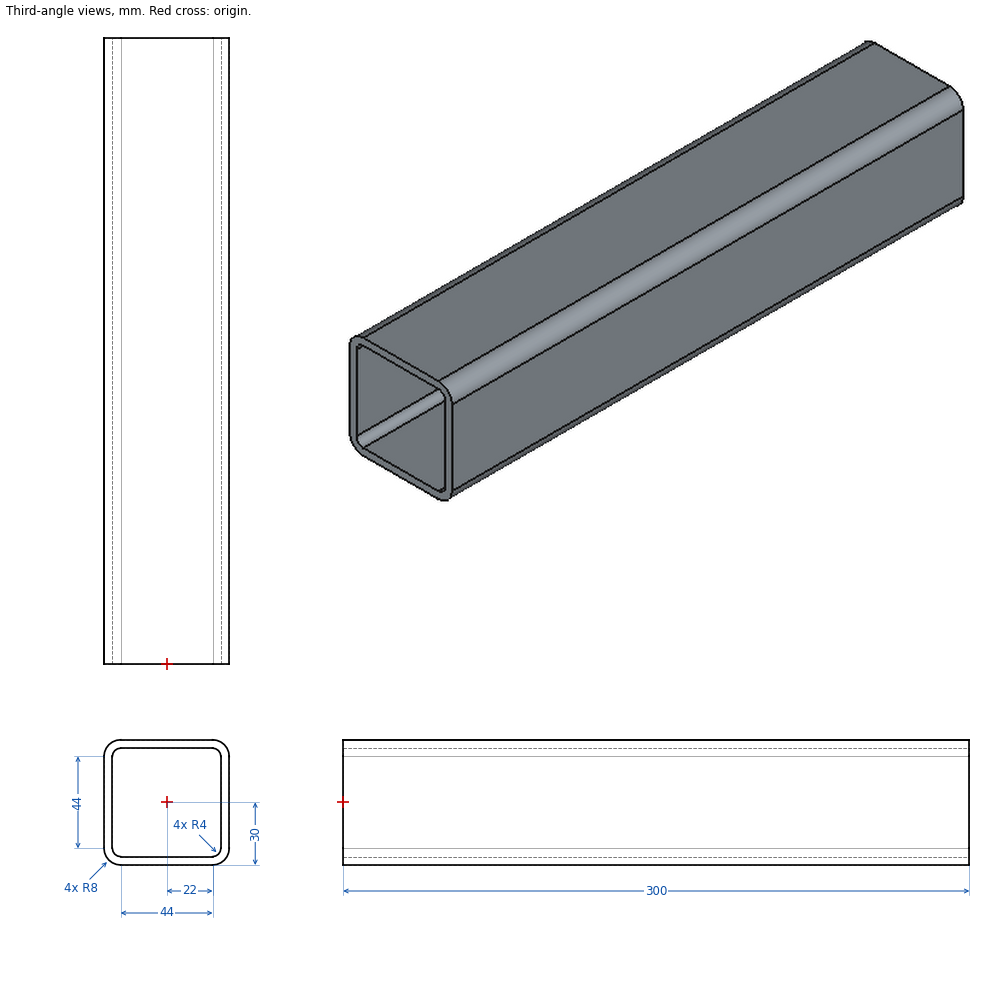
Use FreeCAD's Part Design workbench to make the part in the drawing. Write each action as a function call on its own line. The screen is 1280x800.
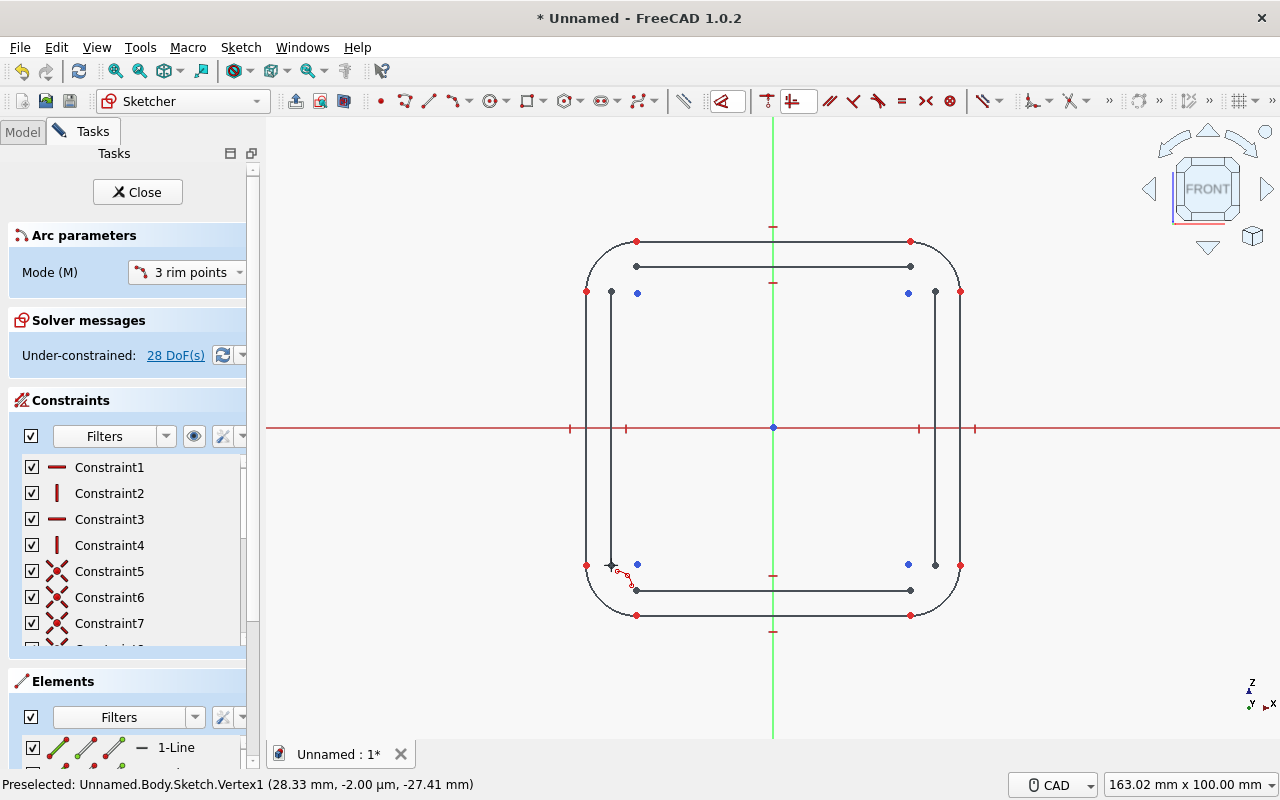
click(910, 591)
click(935, 566)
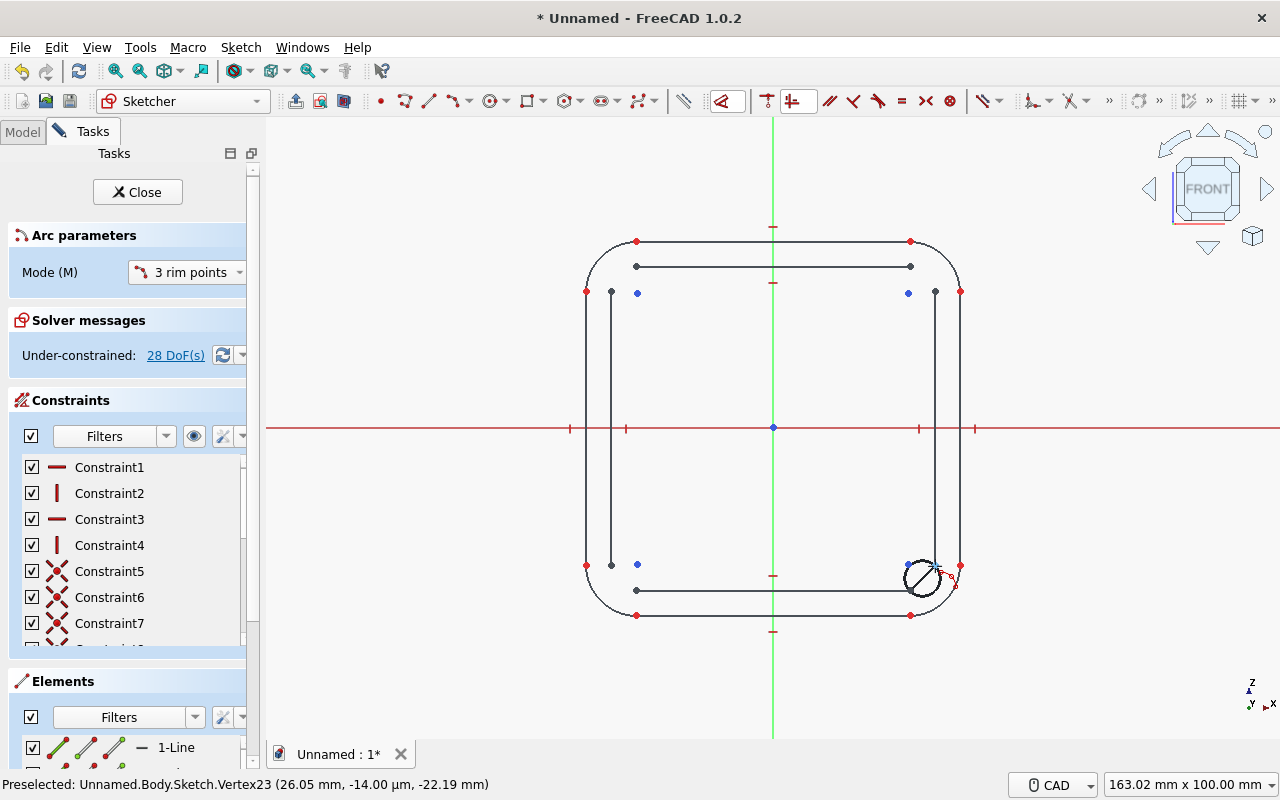
scroll(927, 582, up, 4)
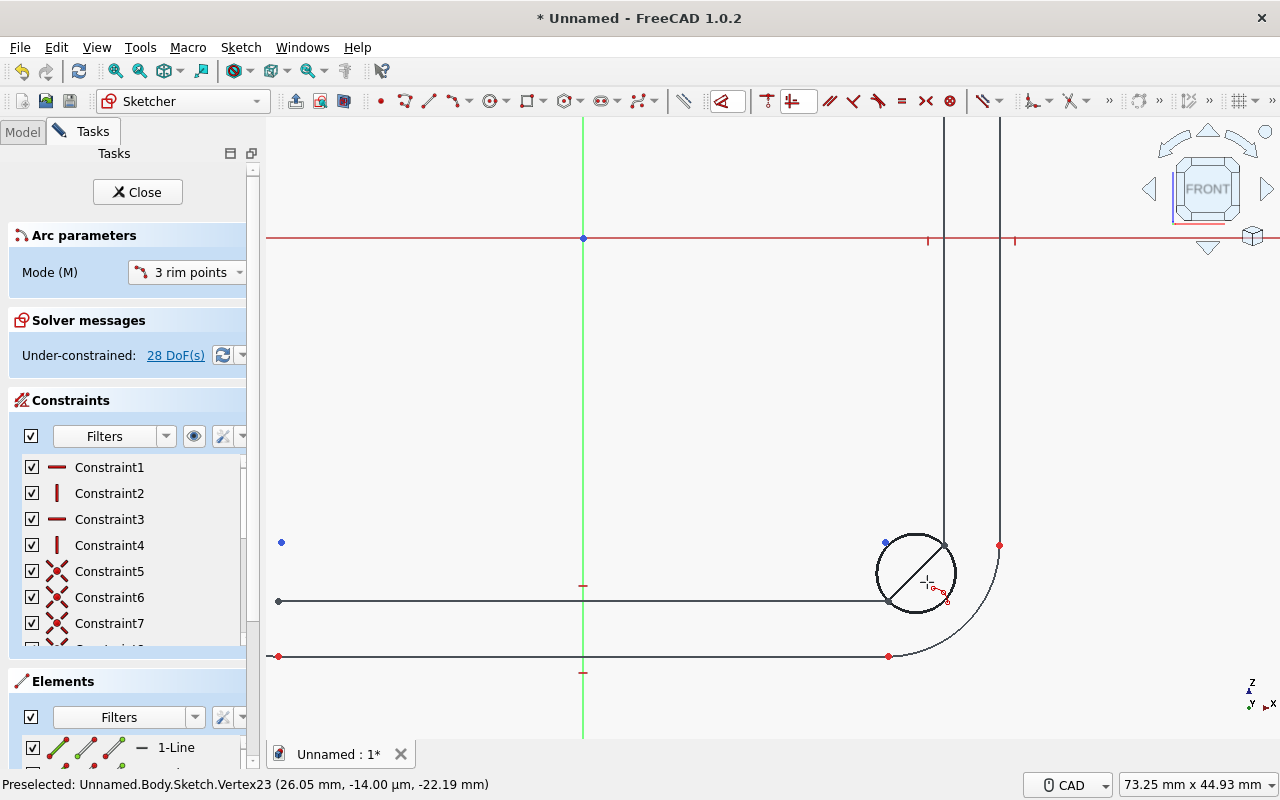
click(927, 582)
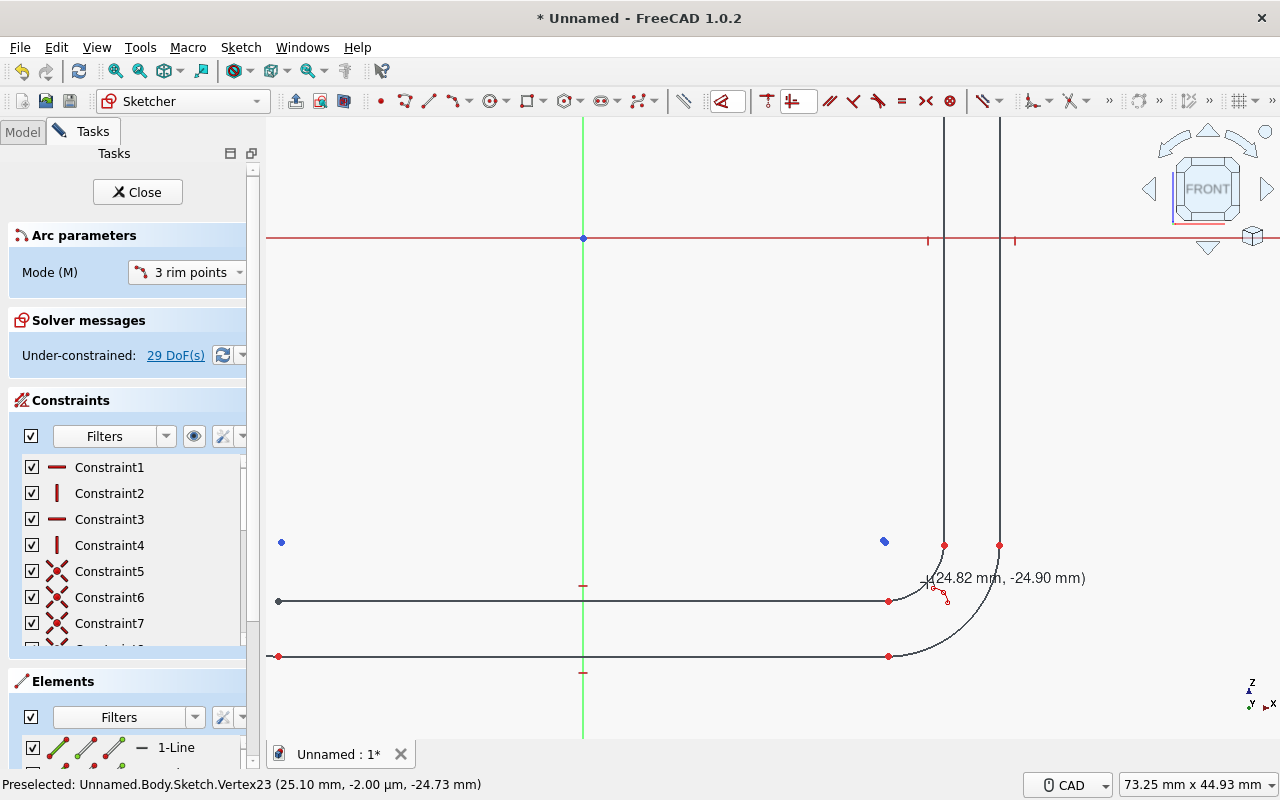
scroll(803, 583, down, 4)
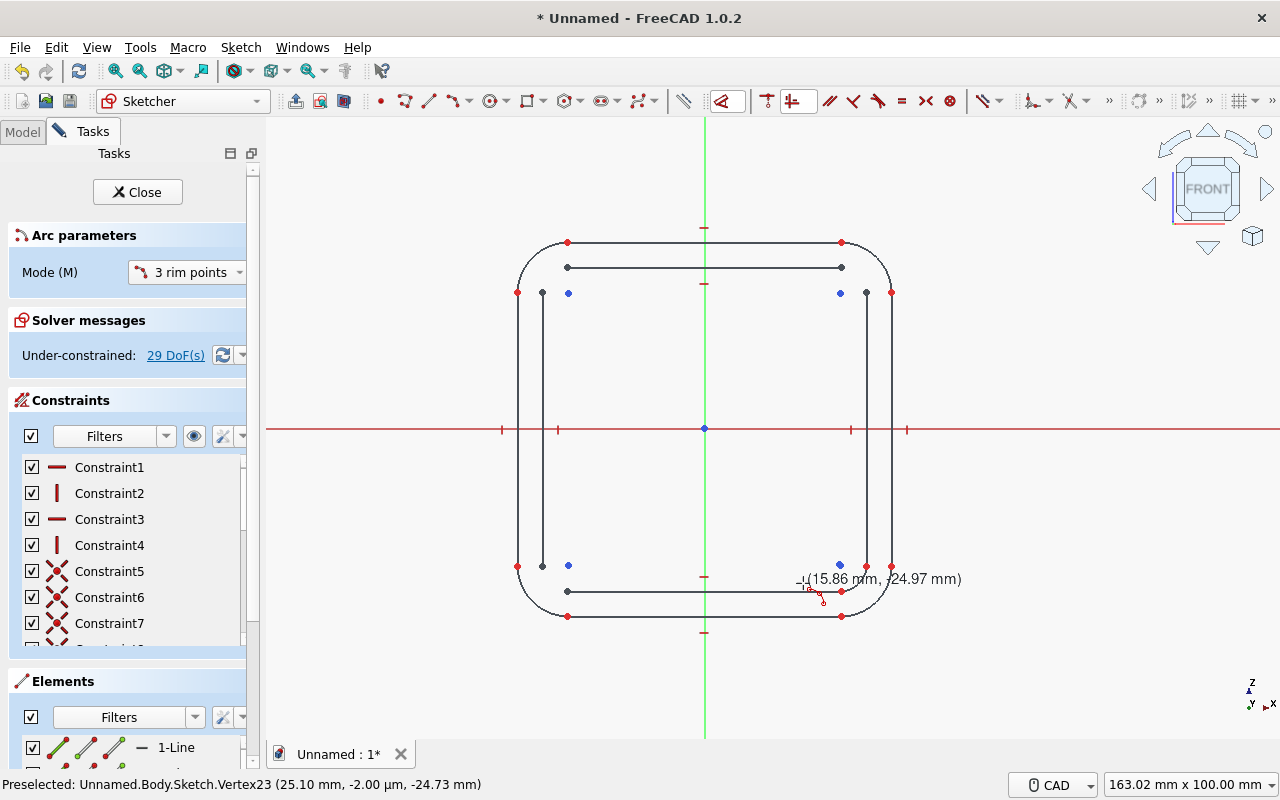
click(867, 293)
click(842, 268)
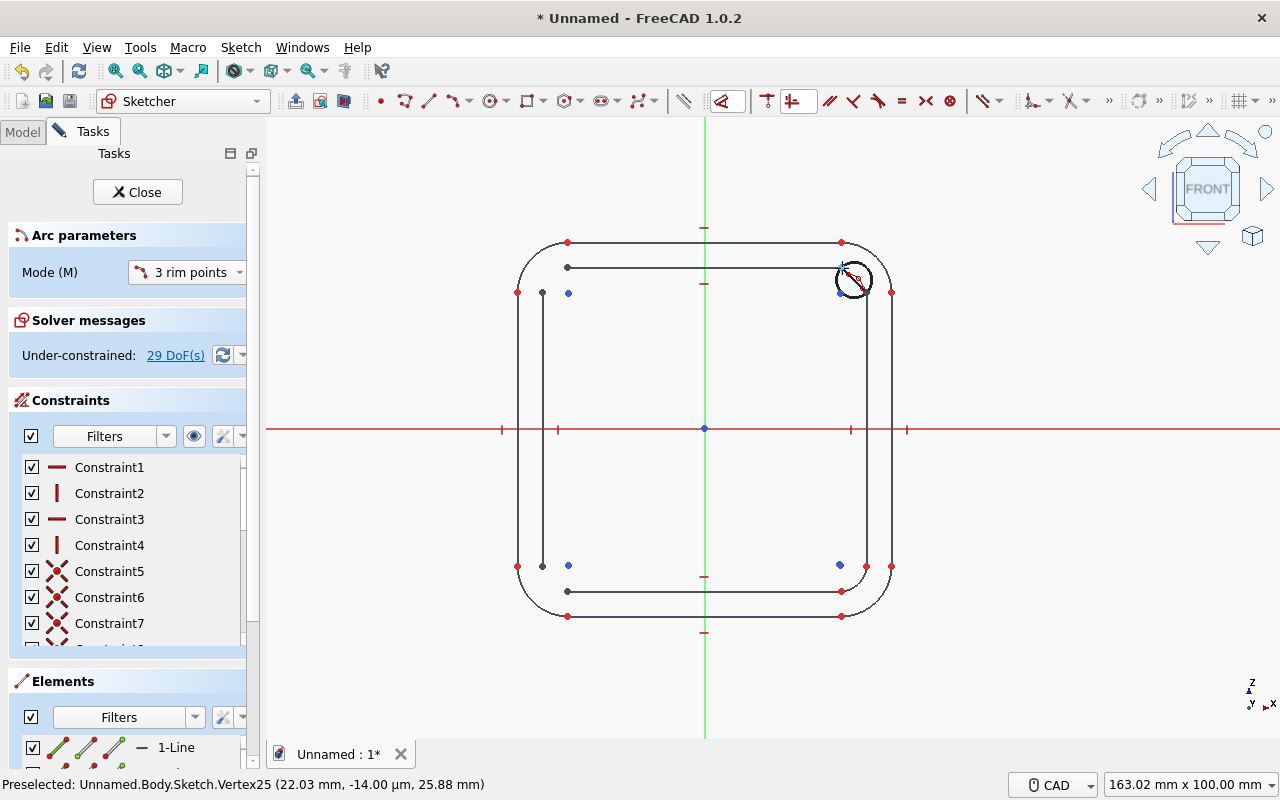
scroll(859, 274, up, 4)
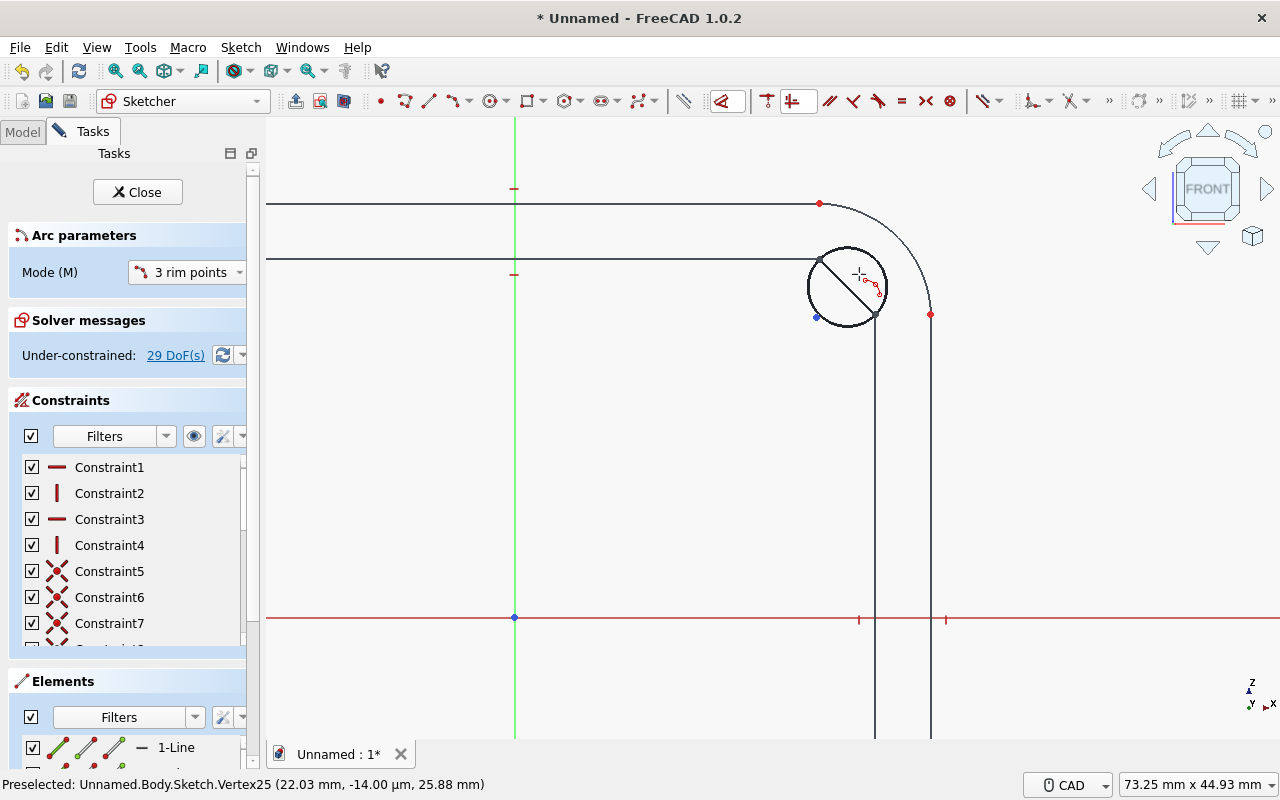
click(858, 274)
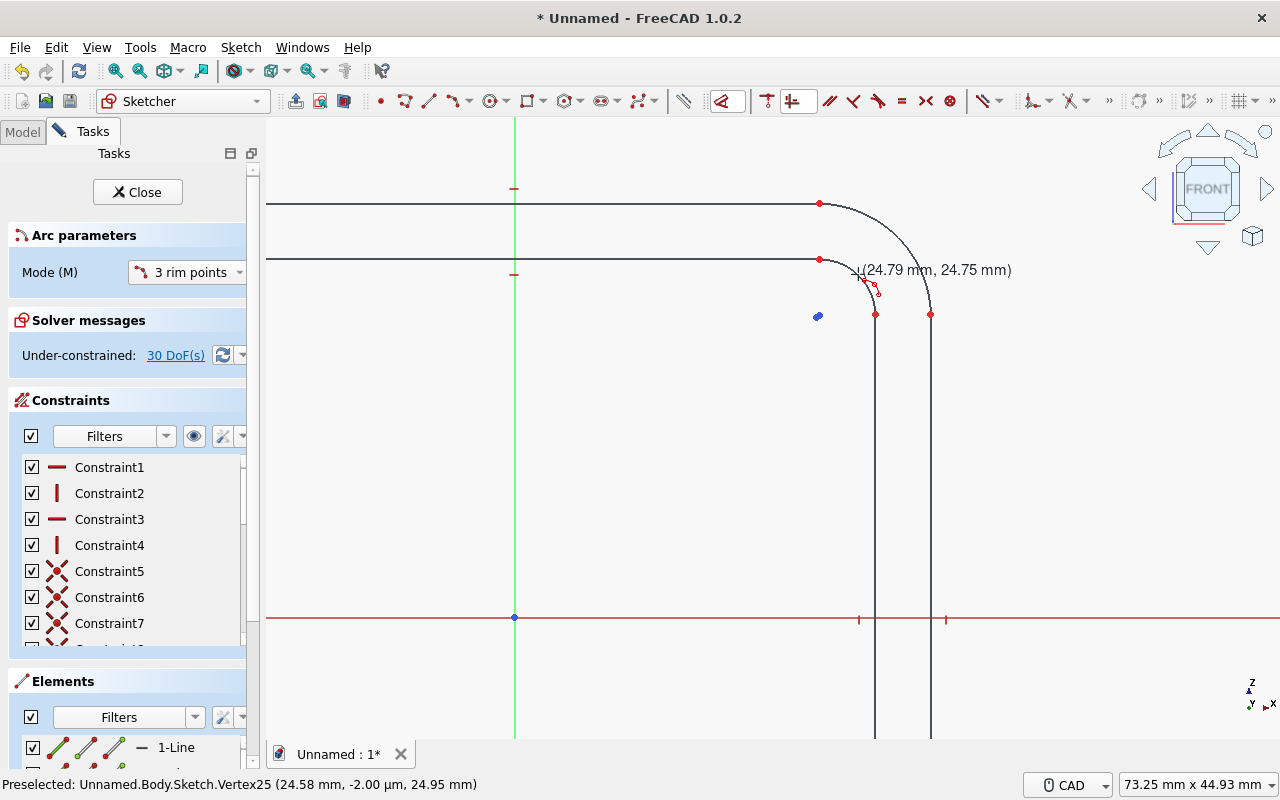
scroll(859, 273, down, 4)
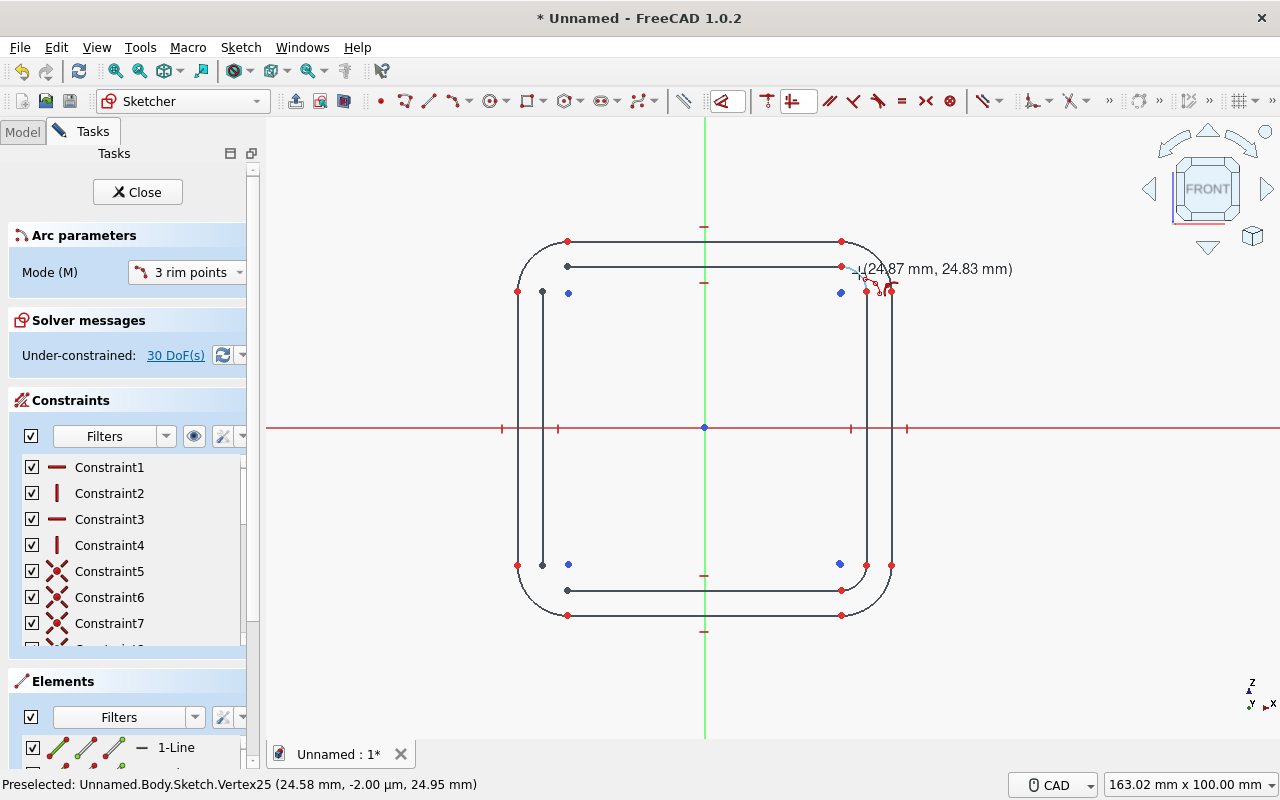
click(568, 267)
click(543, 292)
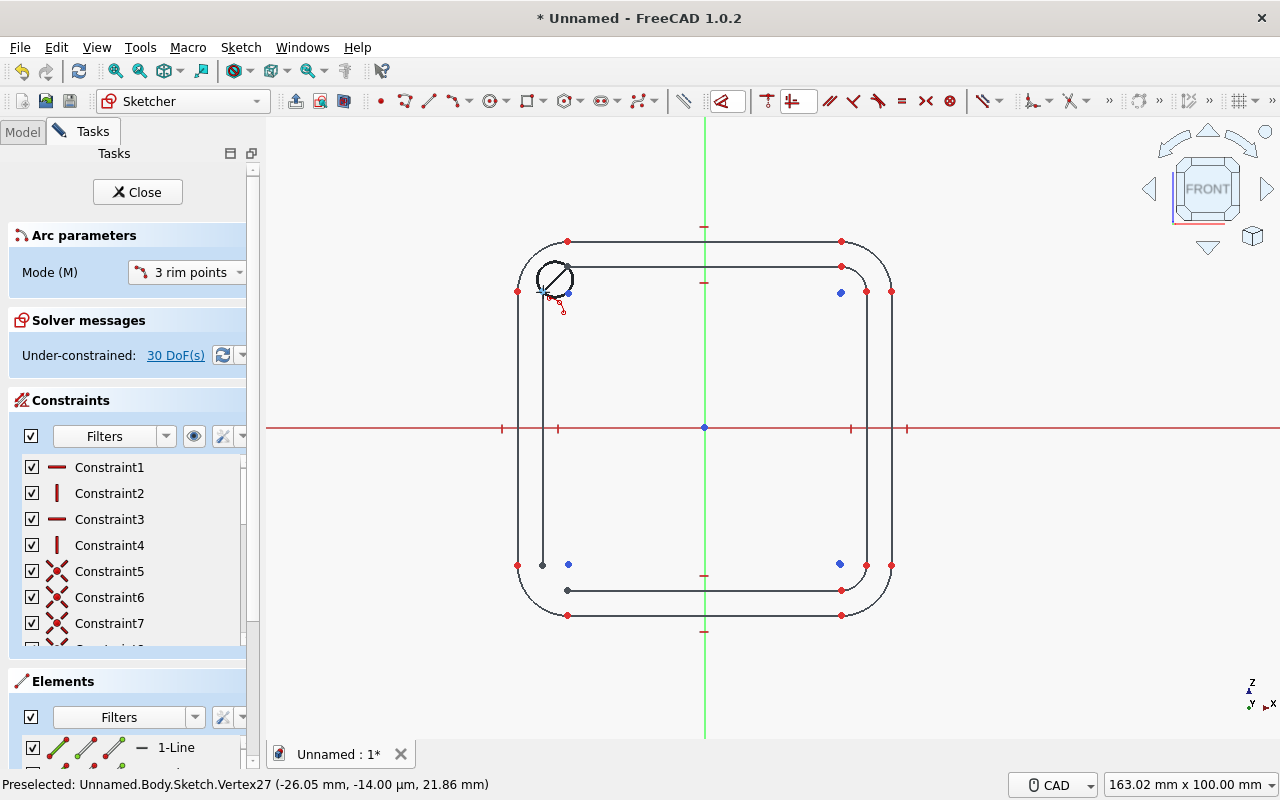
scroll(550, 274, up, 4)